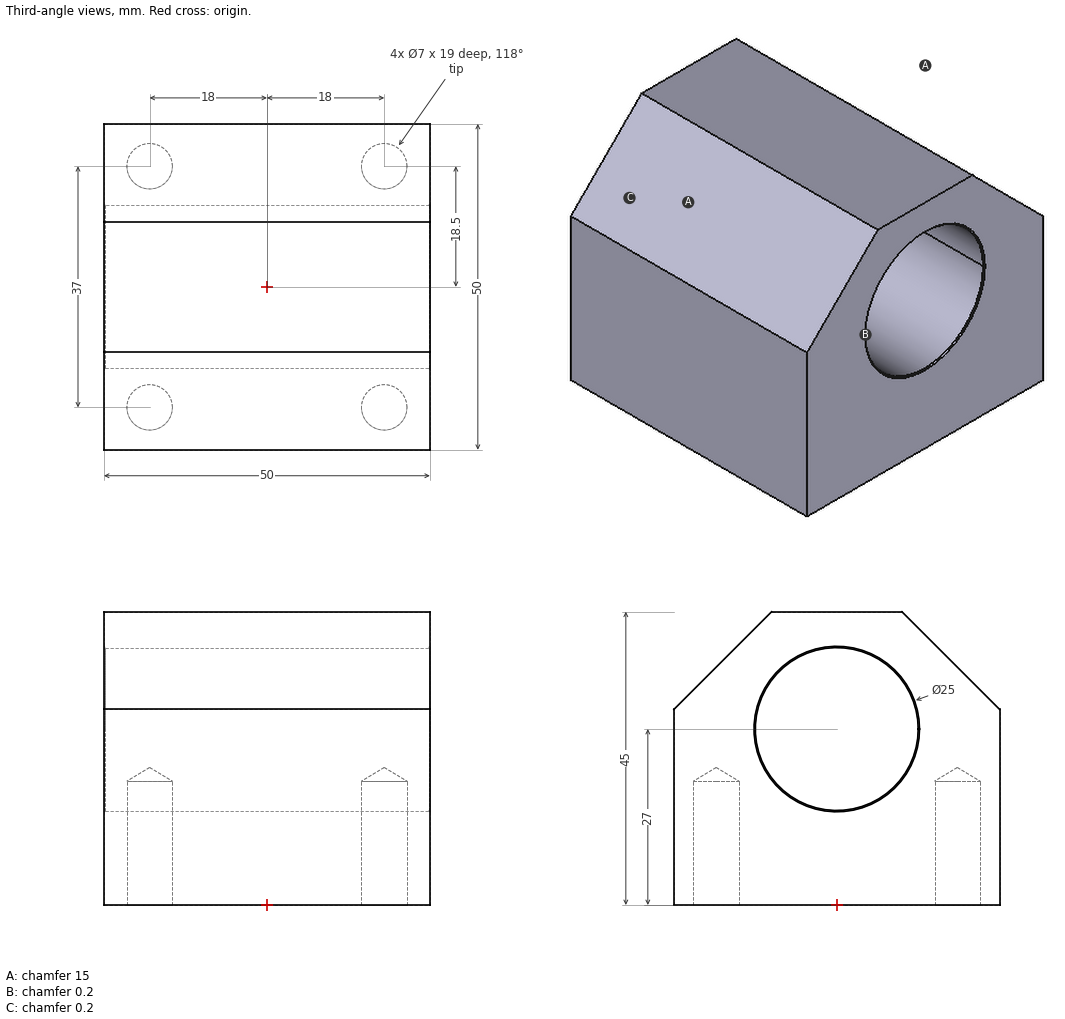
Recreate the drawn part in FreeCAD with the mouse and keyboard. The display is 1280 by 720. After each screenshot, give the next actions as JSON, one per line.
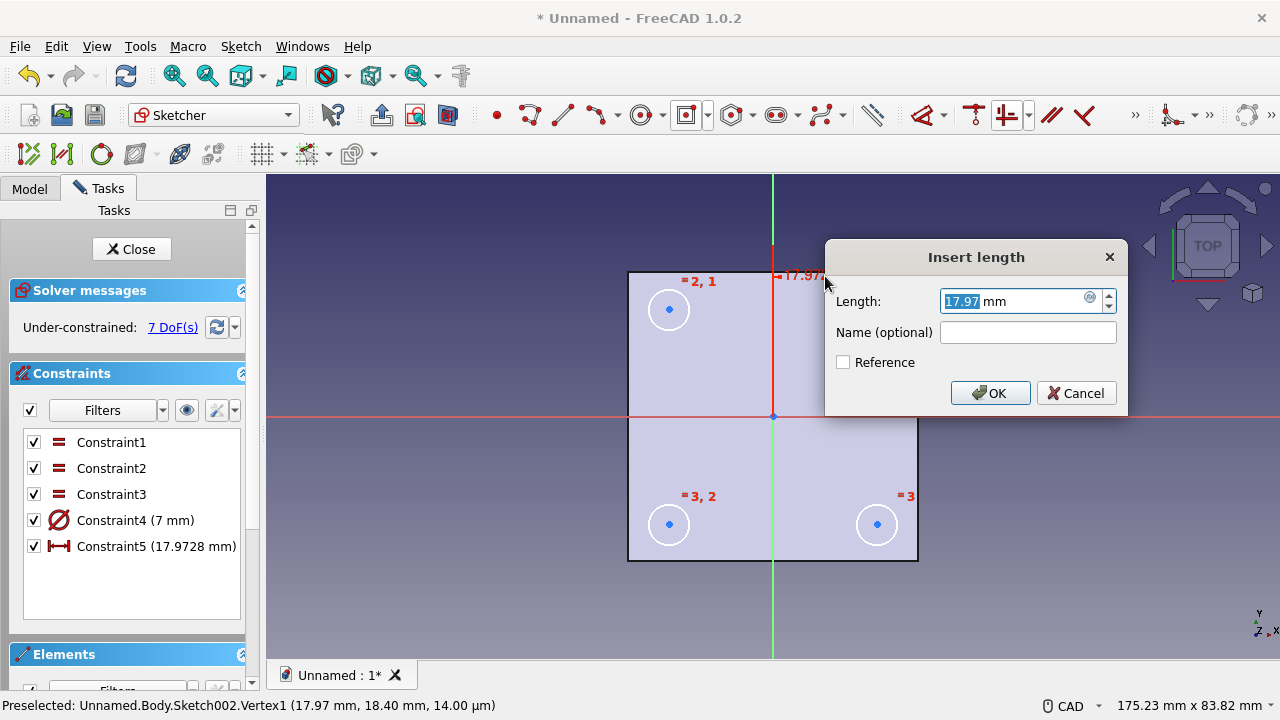
{"action": "type", "text": "18"}
{"action": "key", "text": "Return"}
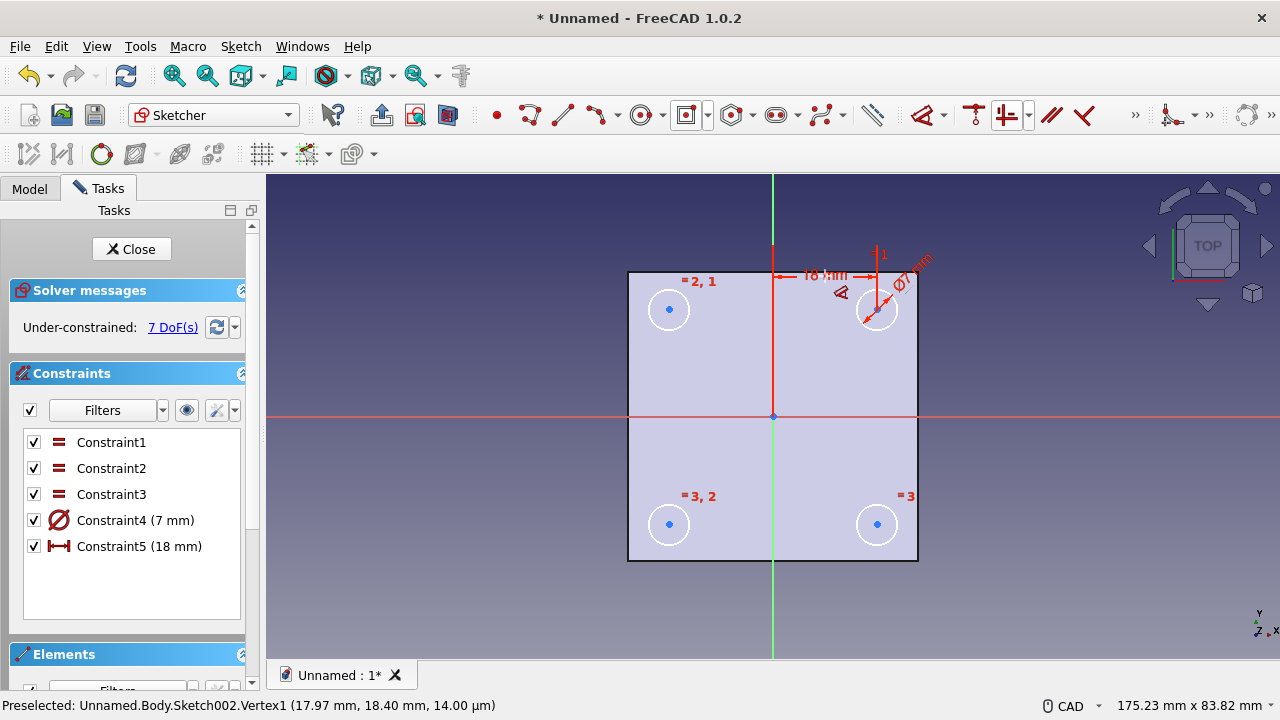
{"action": "left_click", "coordinate": [669, 310]}
{"action": "left_click", "coordinate": [721, 276]}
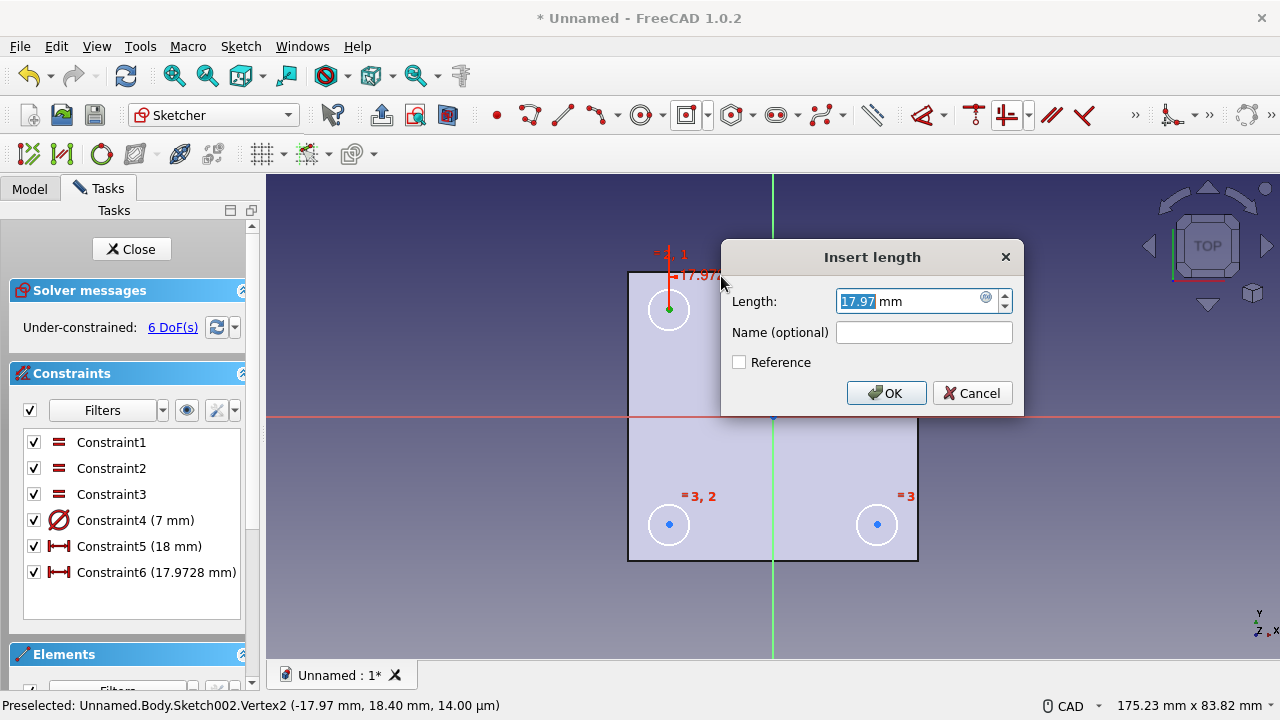
{"action": "type", "text": "18"}
{"action": "key", "text": "Return"}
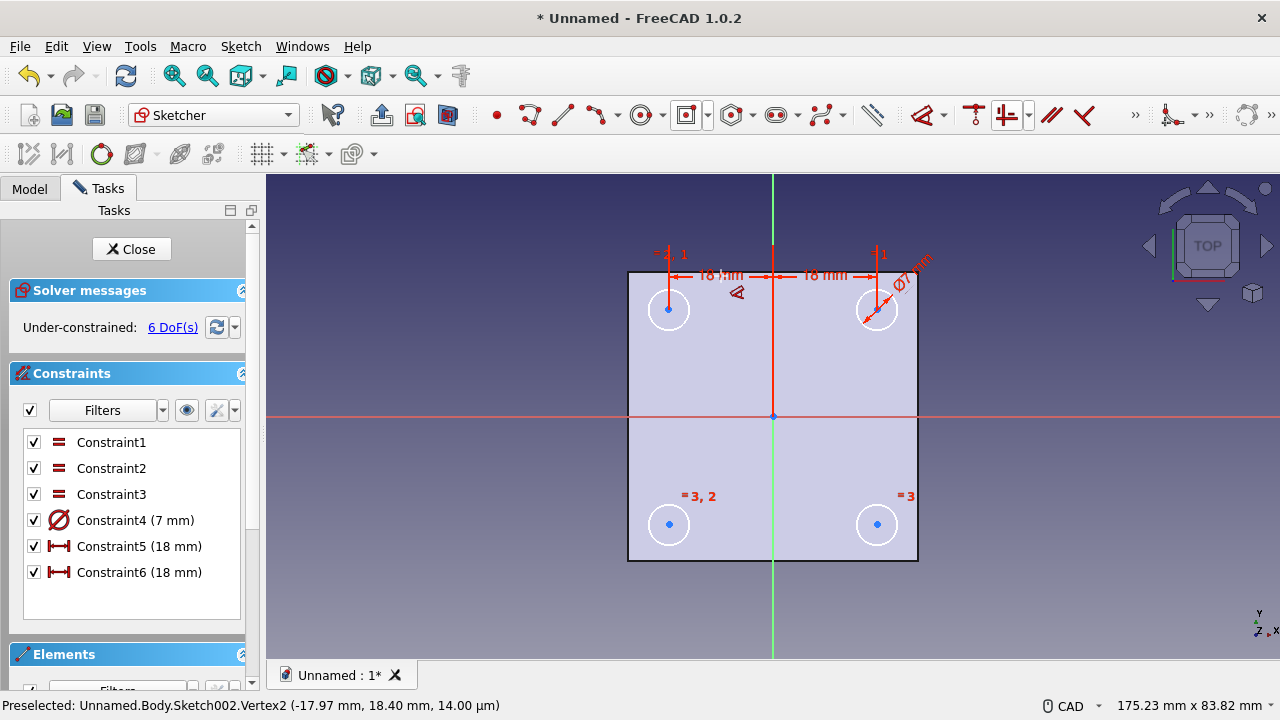
{"action": "left_click", "coordinate": [669, 525]}
{"action": "left_click", "coordinate": [721, 559]}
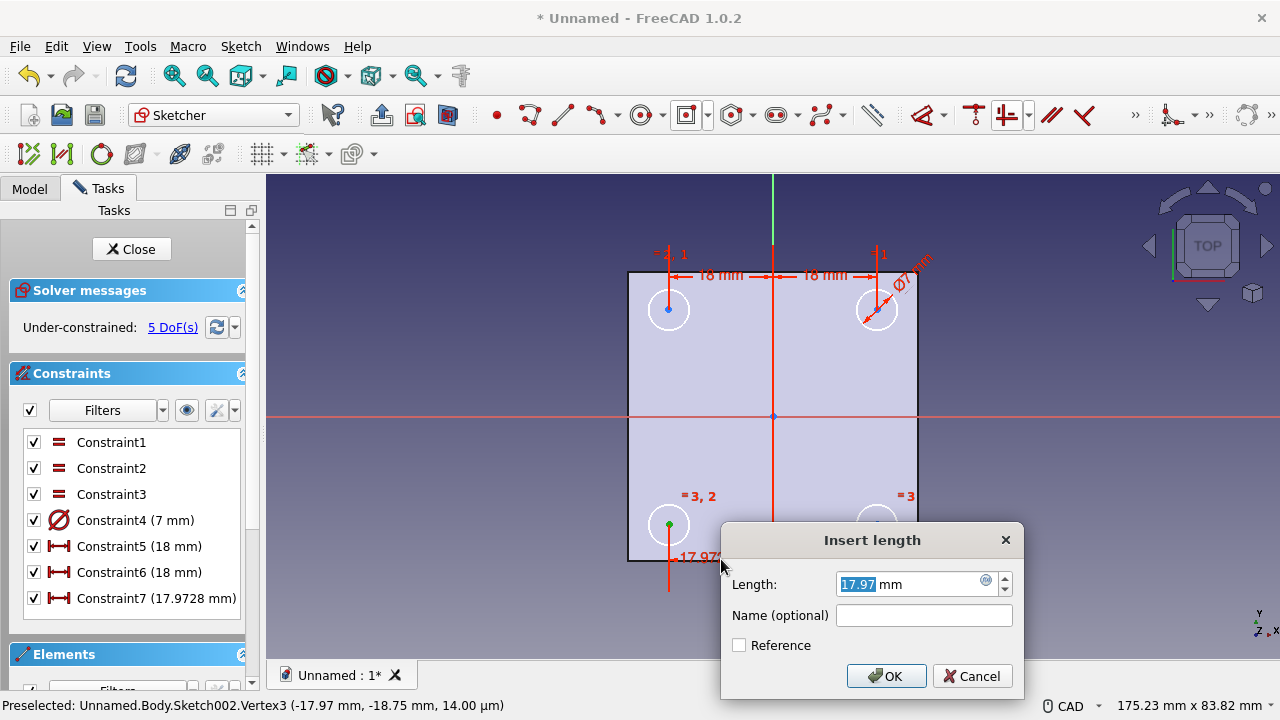
{"action": "type", "text": "18"}
{"action": "key", "text": "Return"}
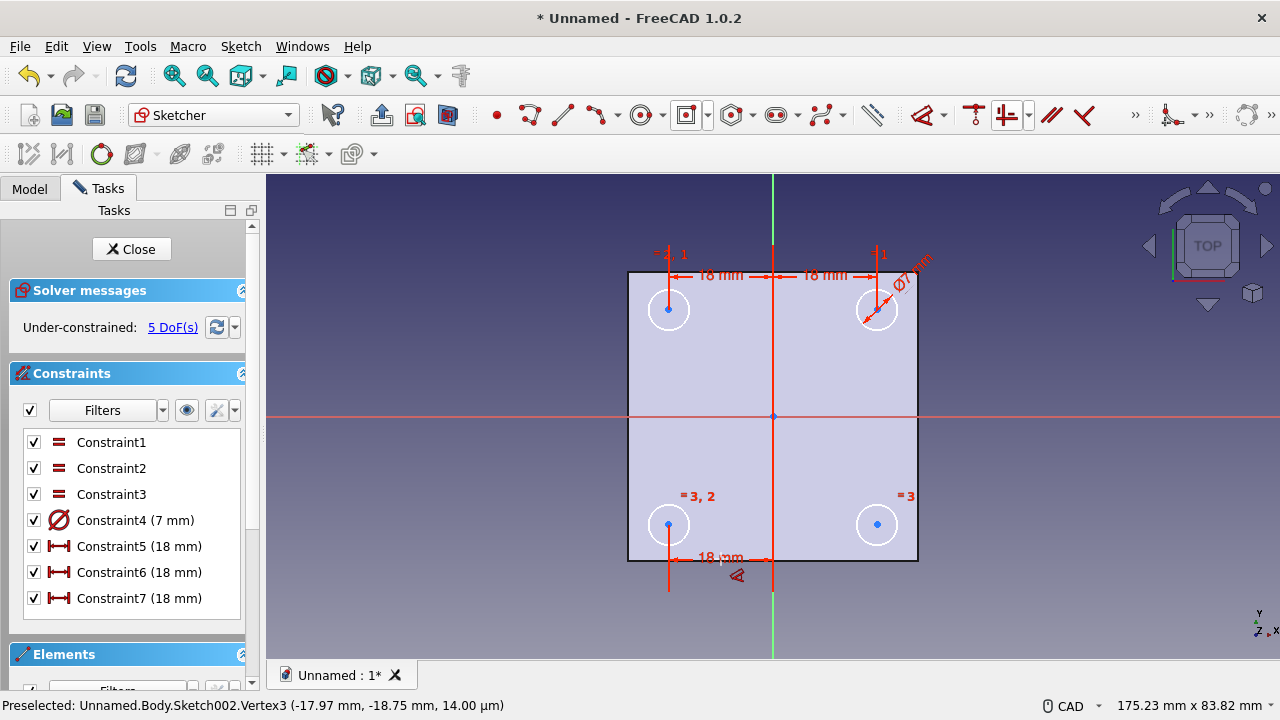
{"action": "left_click", "coordinate": [877, 525]}
{"action": "left_click", "coordinate": [825, 559]}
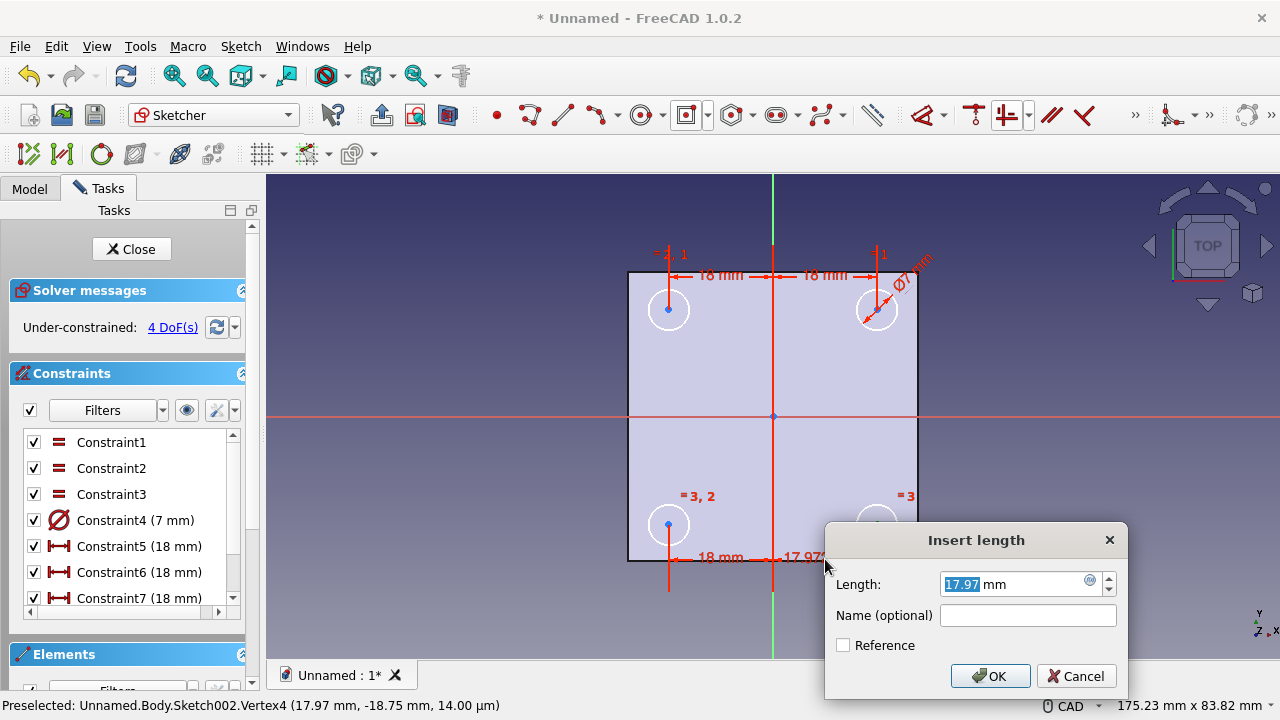
{"action": "type", "text": "18"}
{"action": "key", "text": "Return"}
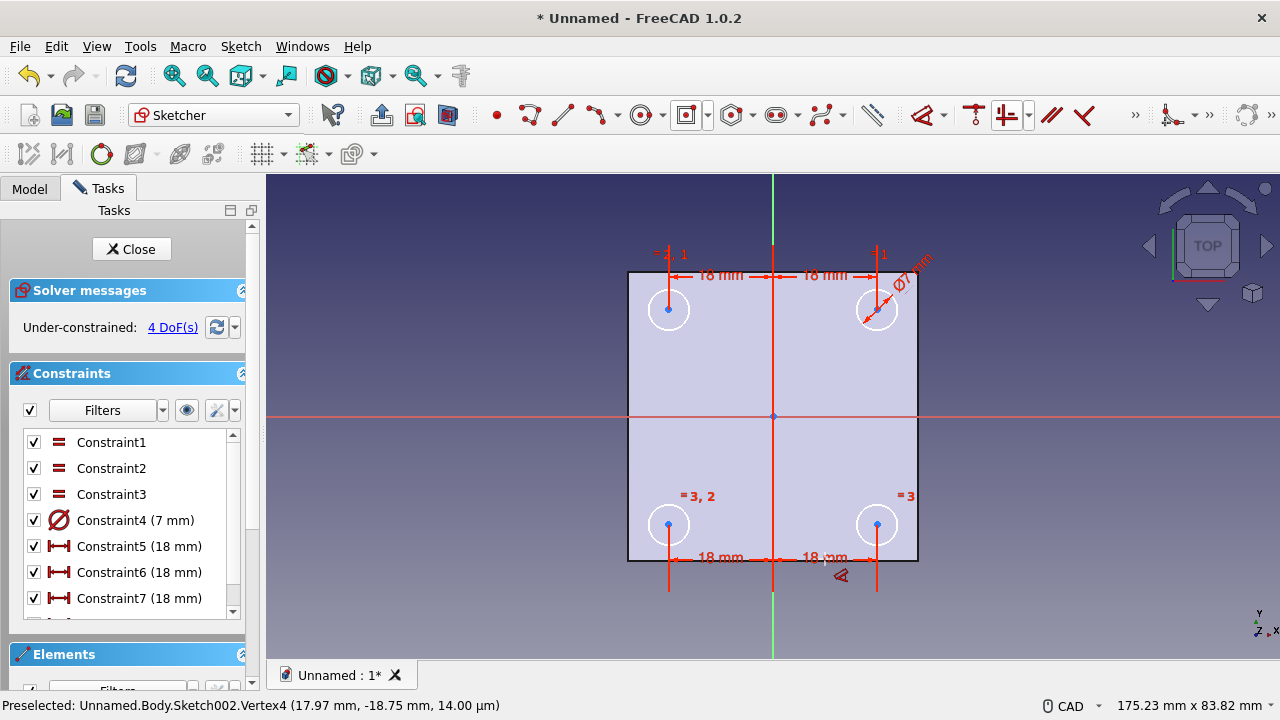
{"action": "left_click", "coordinate": [669, 310]}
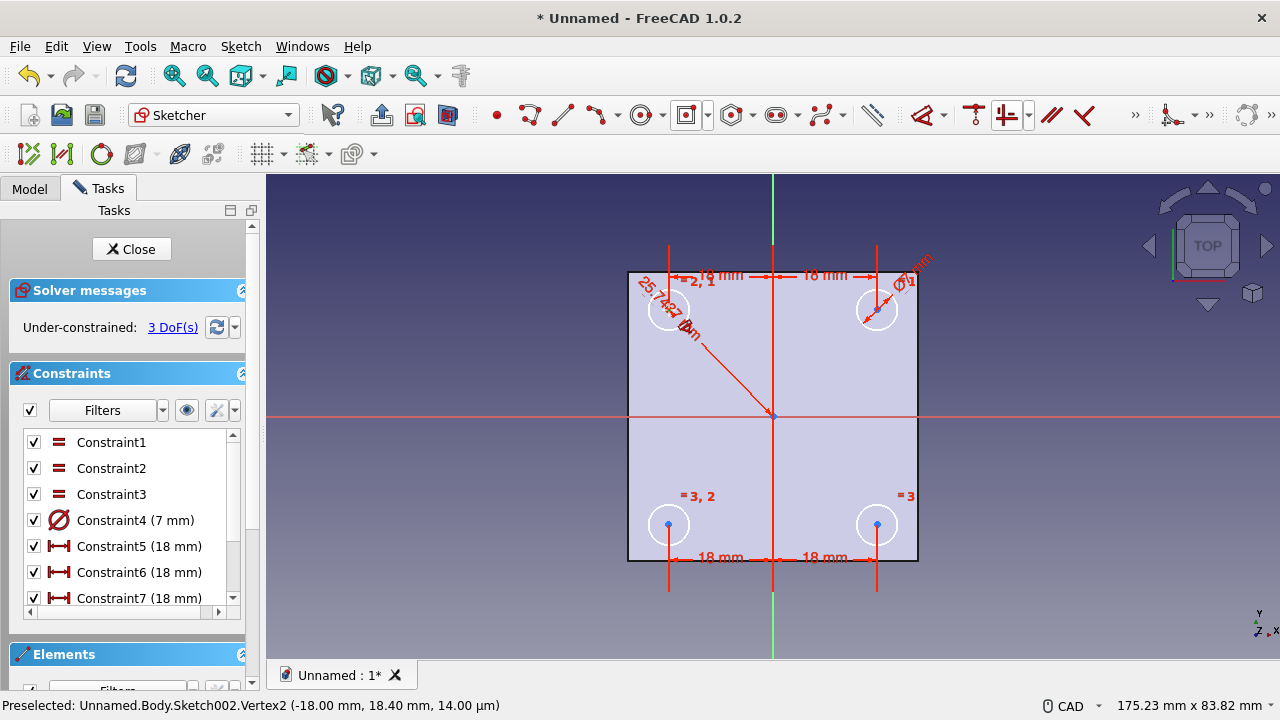
{"action": "left_click", "coordinate": [669, 525]}
{"action": "left_click", "coordinate": [635, 368]}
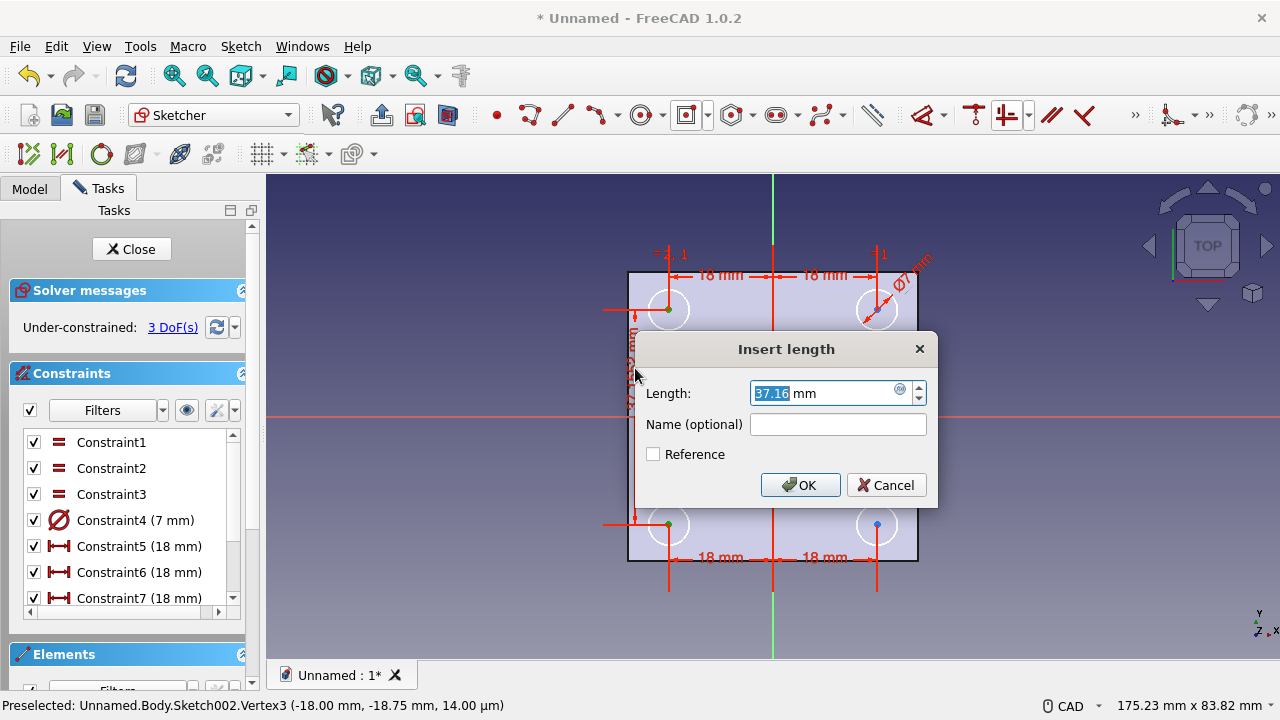
{"action": "type", "text": "37"}
{"action": "key", "text": "Return"}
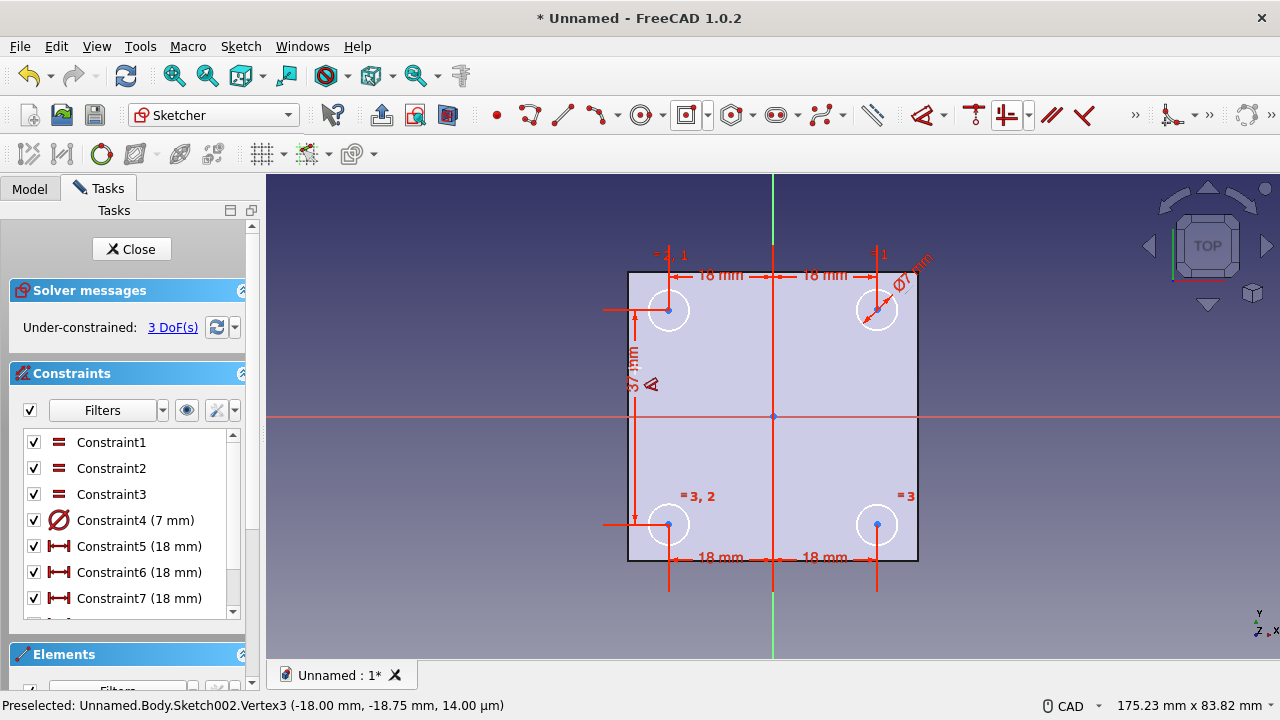
{"action": "left_click", "coordinate": [877, 310]}